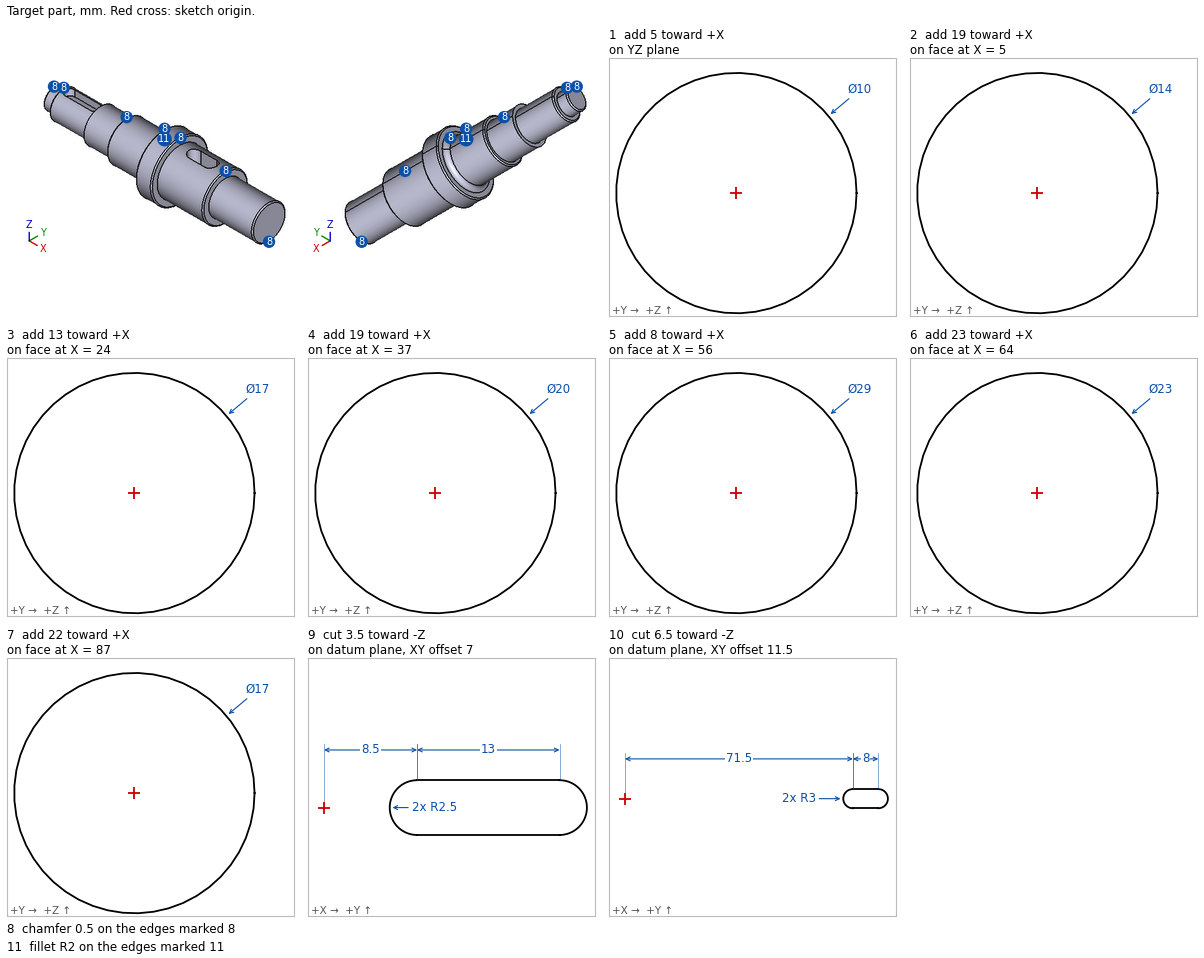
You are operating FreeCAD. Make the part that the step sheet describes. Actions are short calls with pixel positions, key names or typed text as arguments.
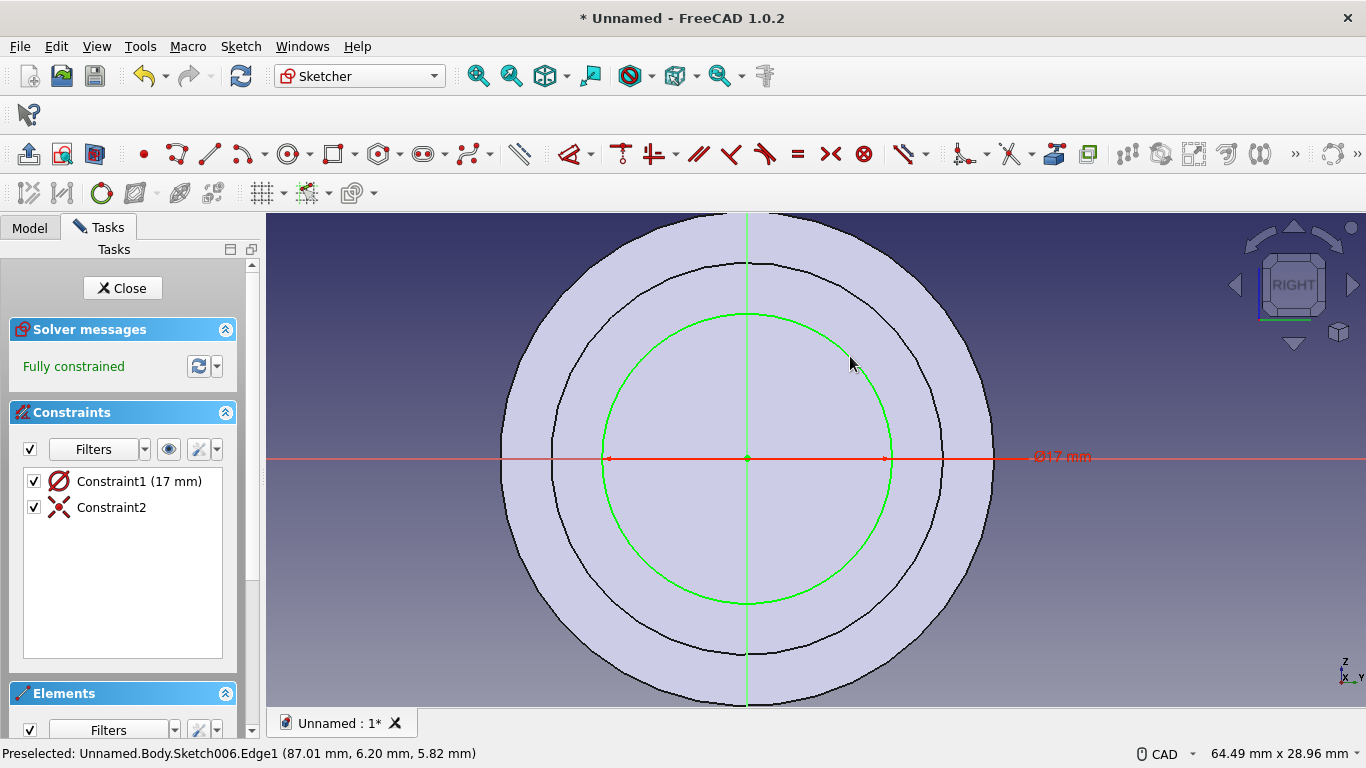
click(123, 288)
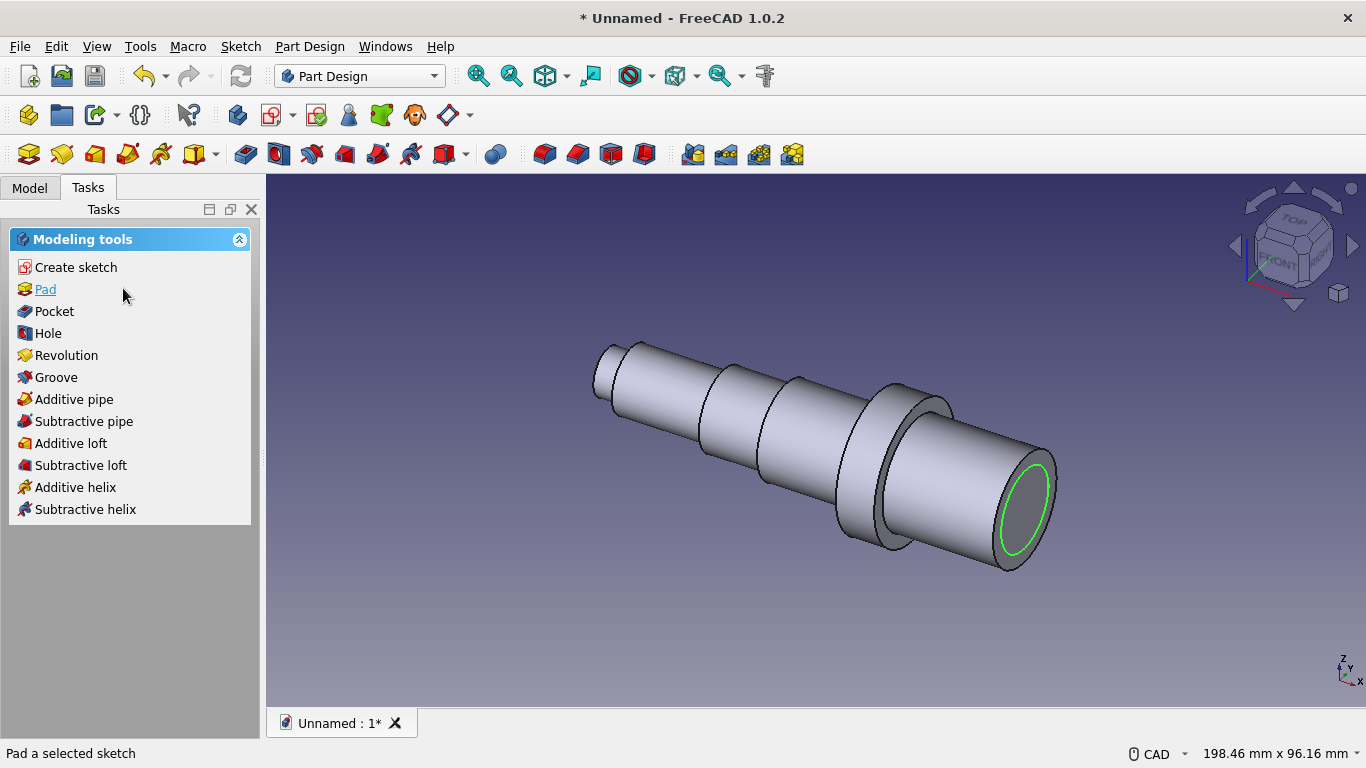
click(29, 154)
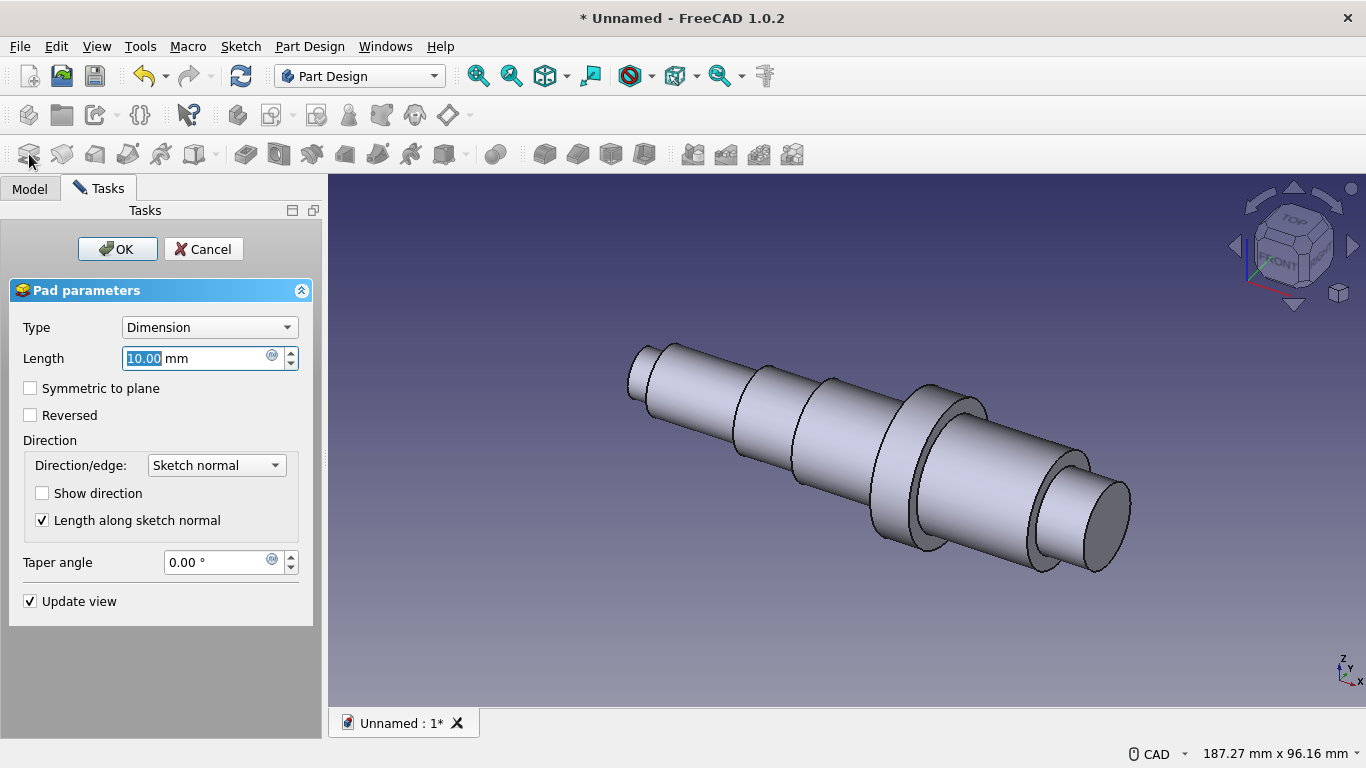
text(22)
key(Tab)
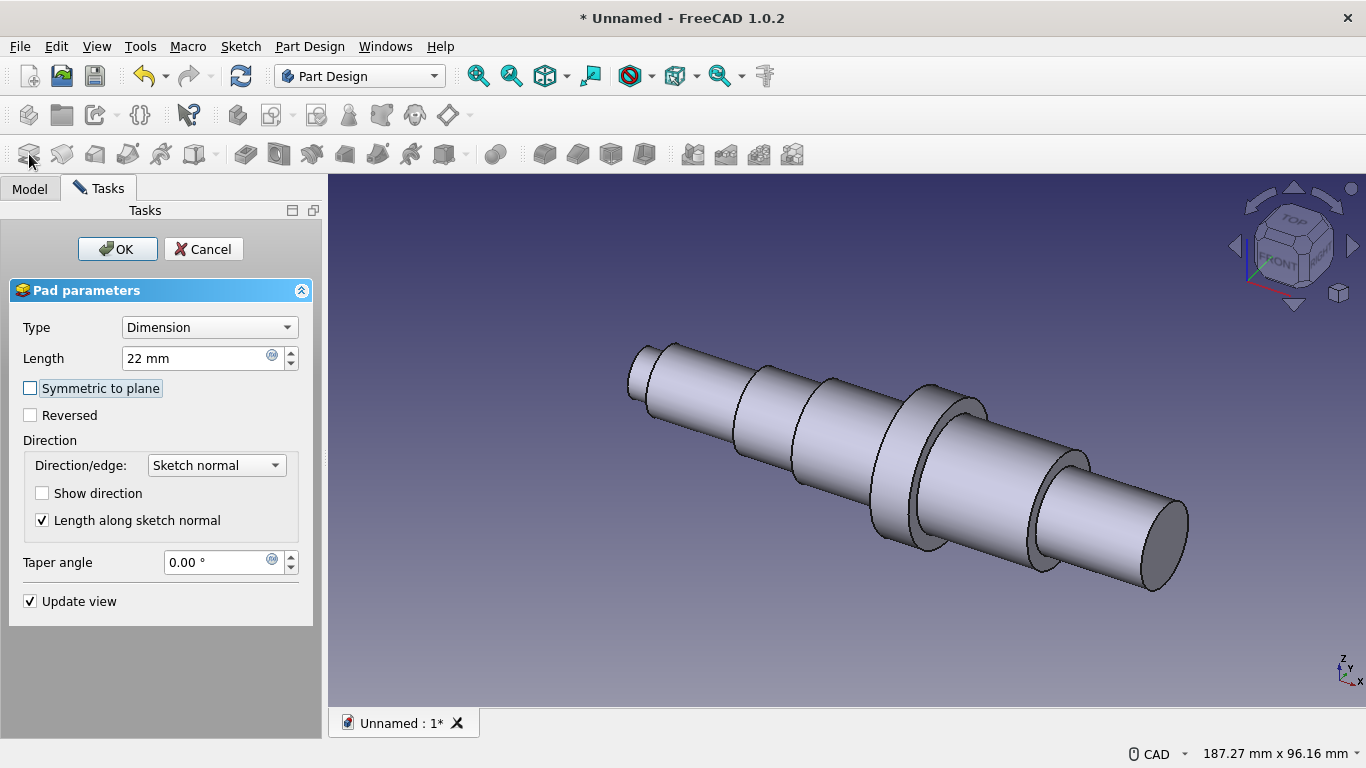
click(118, 249)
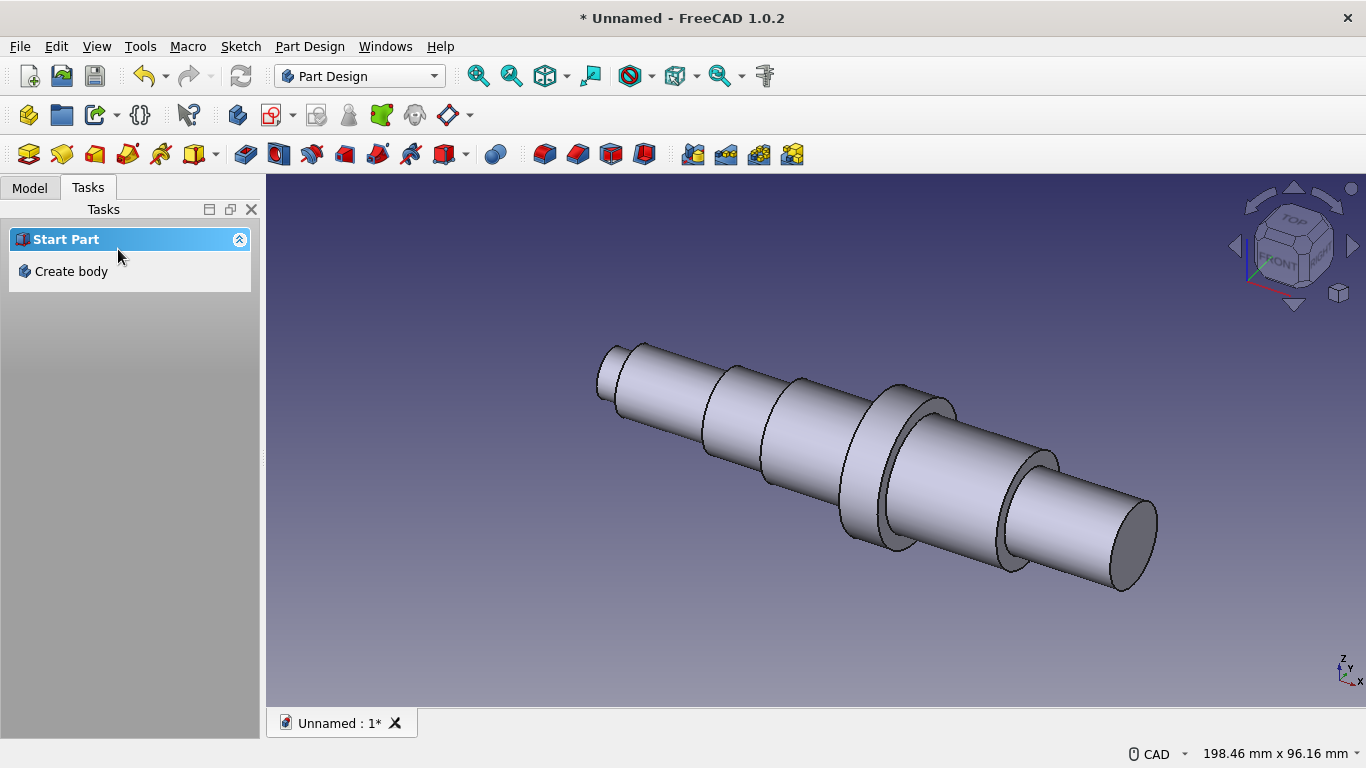
click(867, 410)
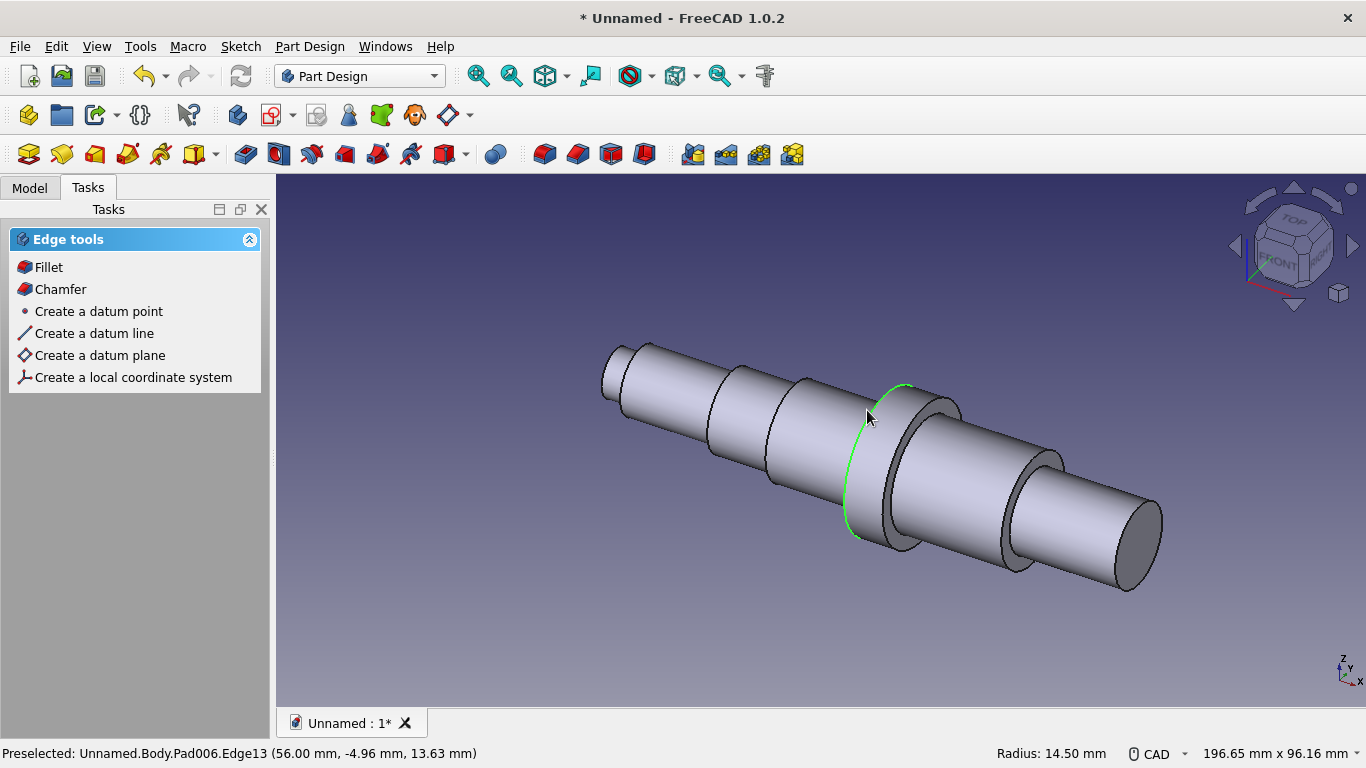
click(620, 346, ctrl)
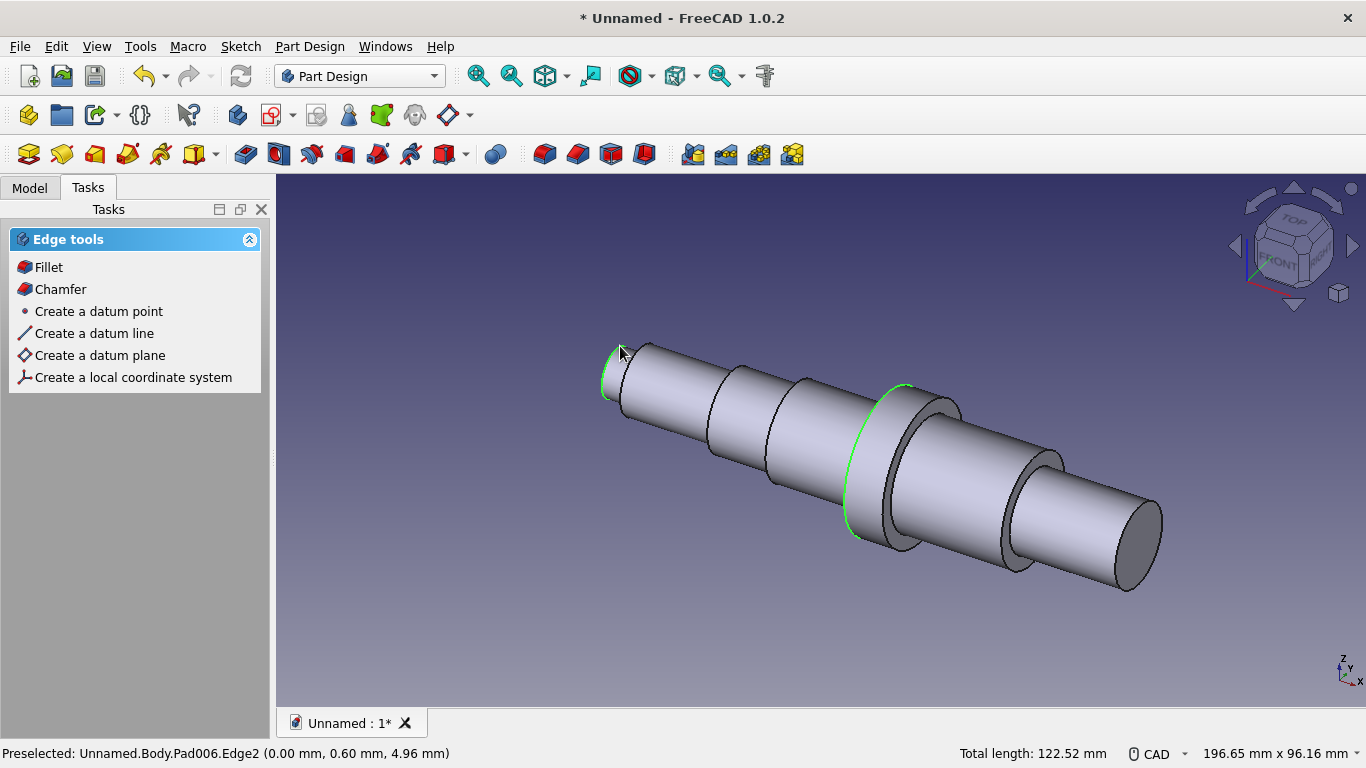
click(882, 513, ctrl)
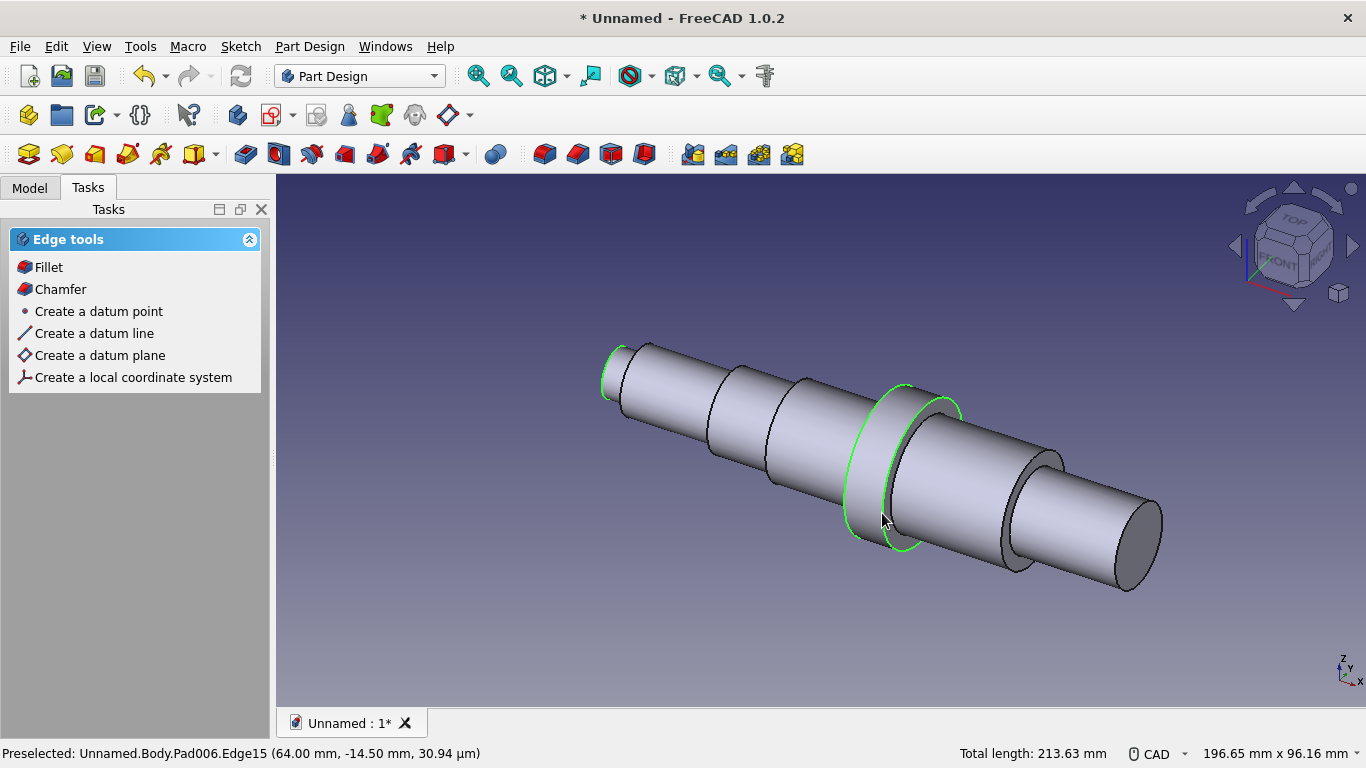
click(1001, 541, ctrl)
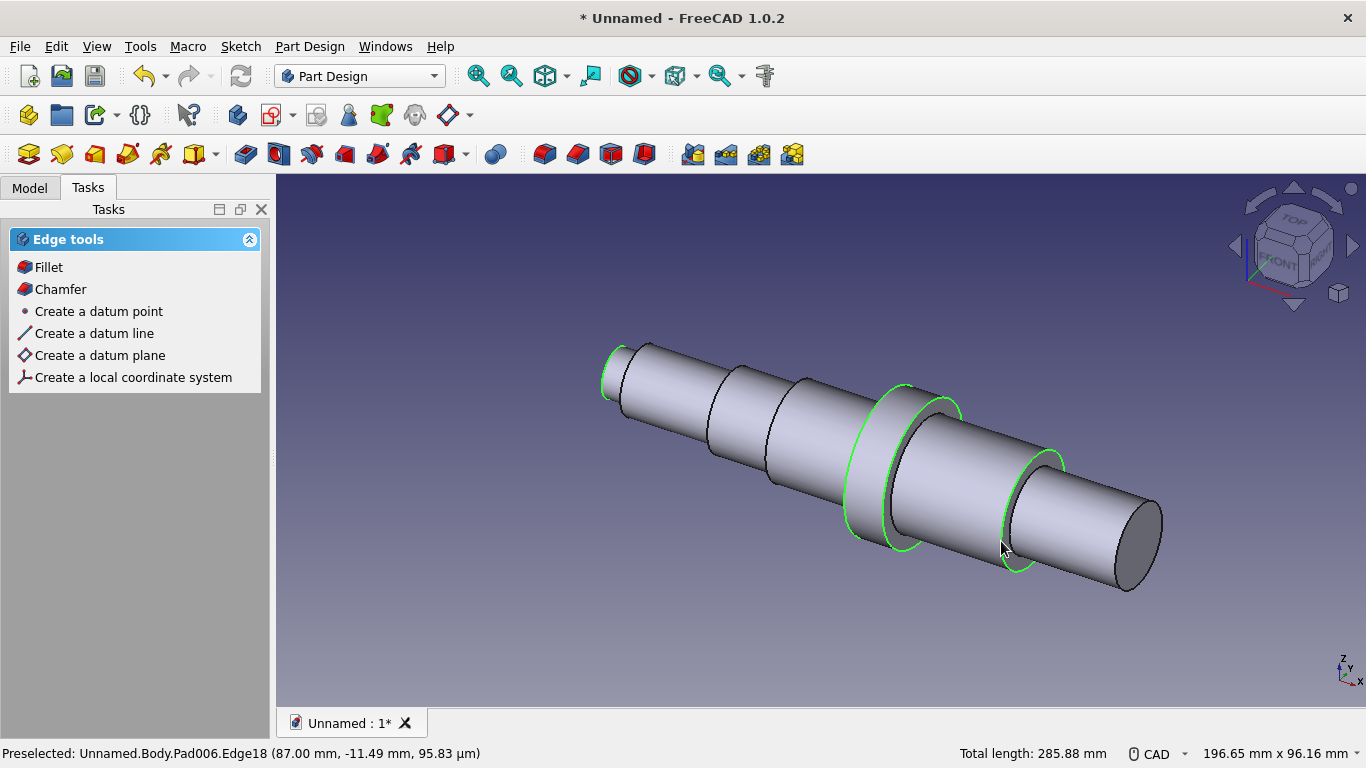
click(1115, 568, ctrl)